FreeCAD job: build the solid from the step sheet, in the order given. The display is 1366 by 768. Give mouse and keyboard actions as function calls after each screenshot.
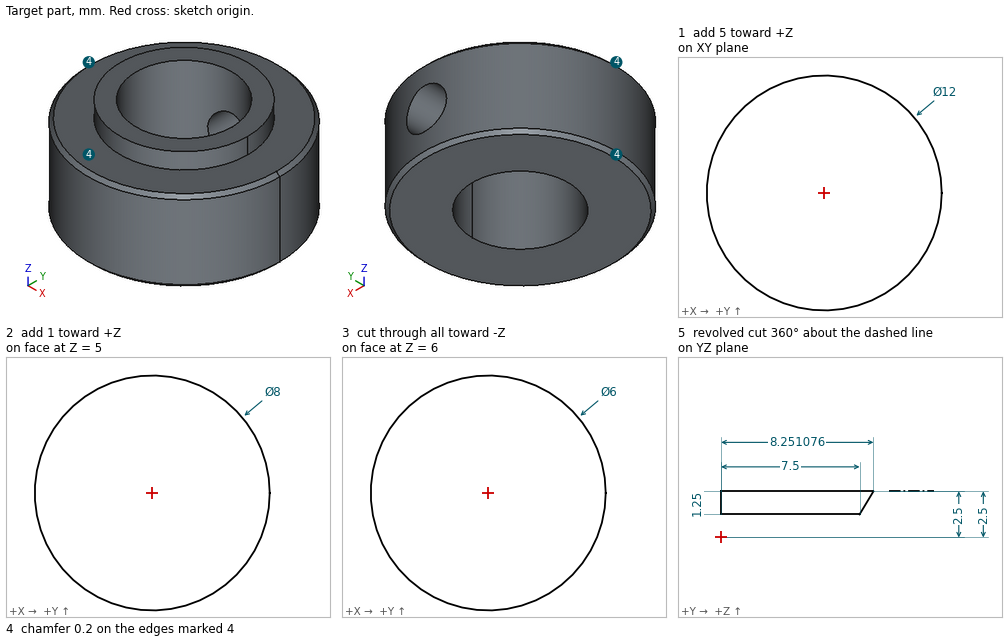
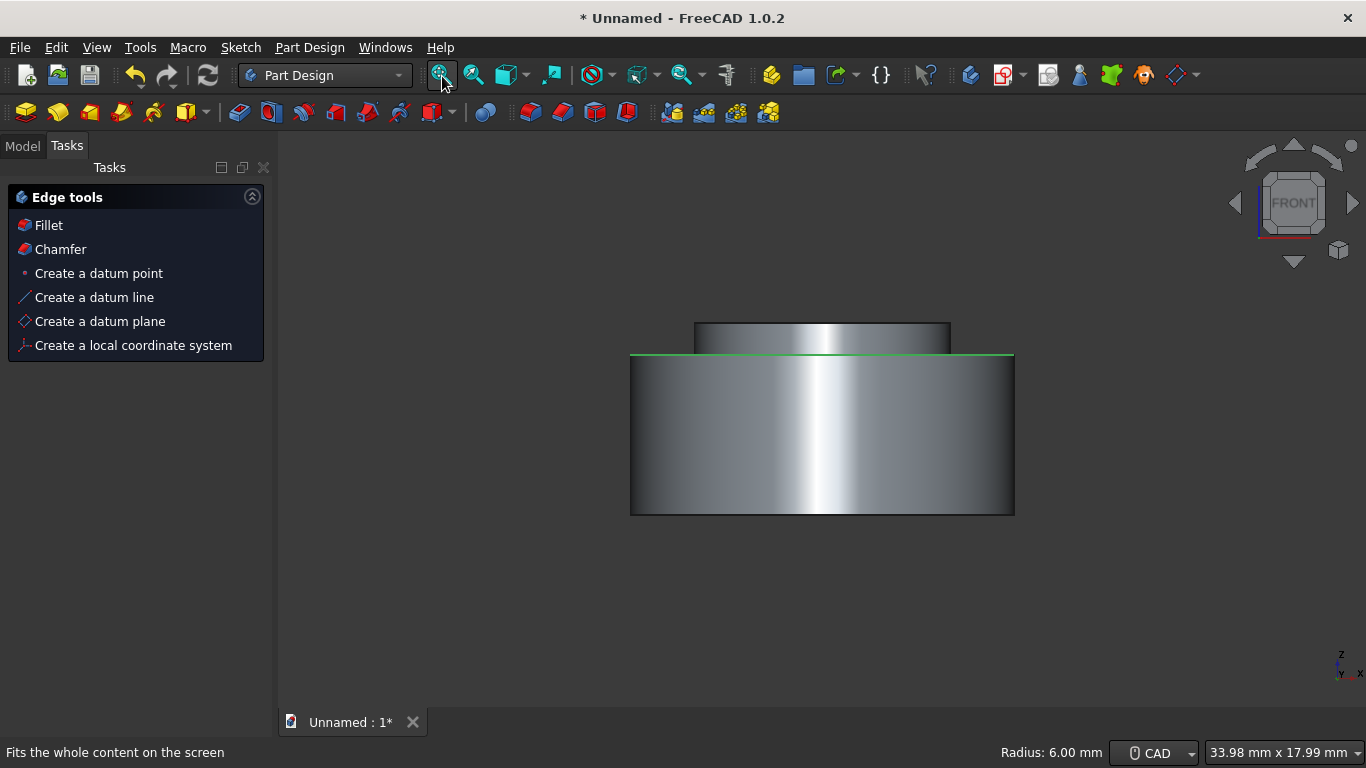
click(666, 514, ctrl)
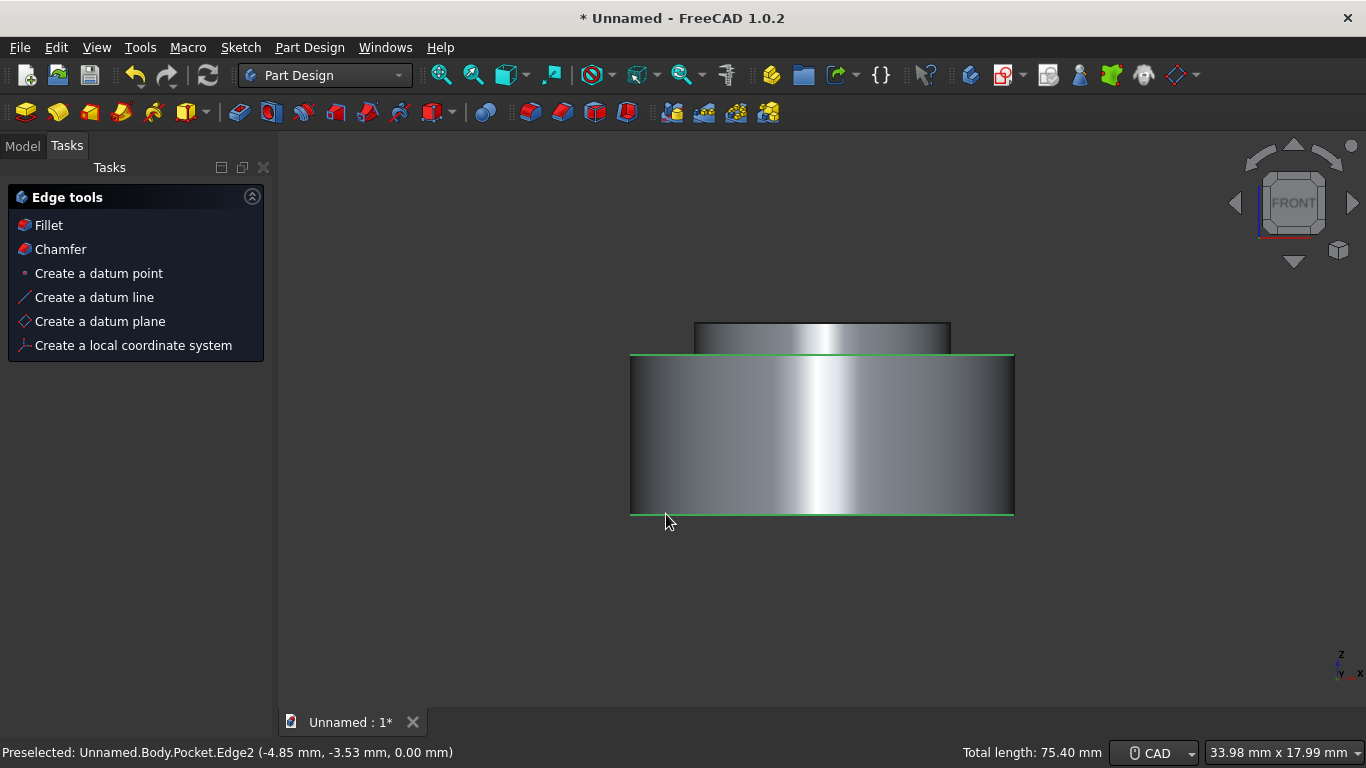
click(564, 112)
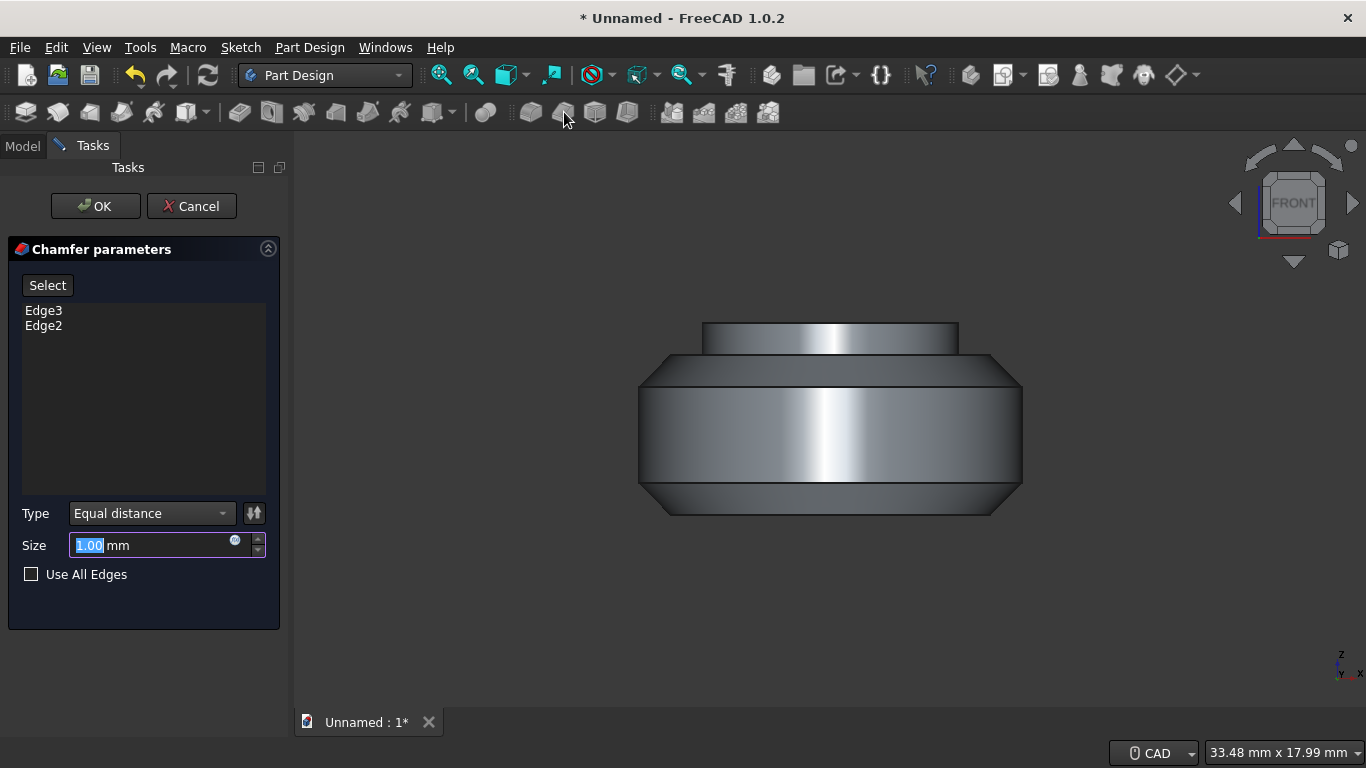
text(0.2)
key(Tab)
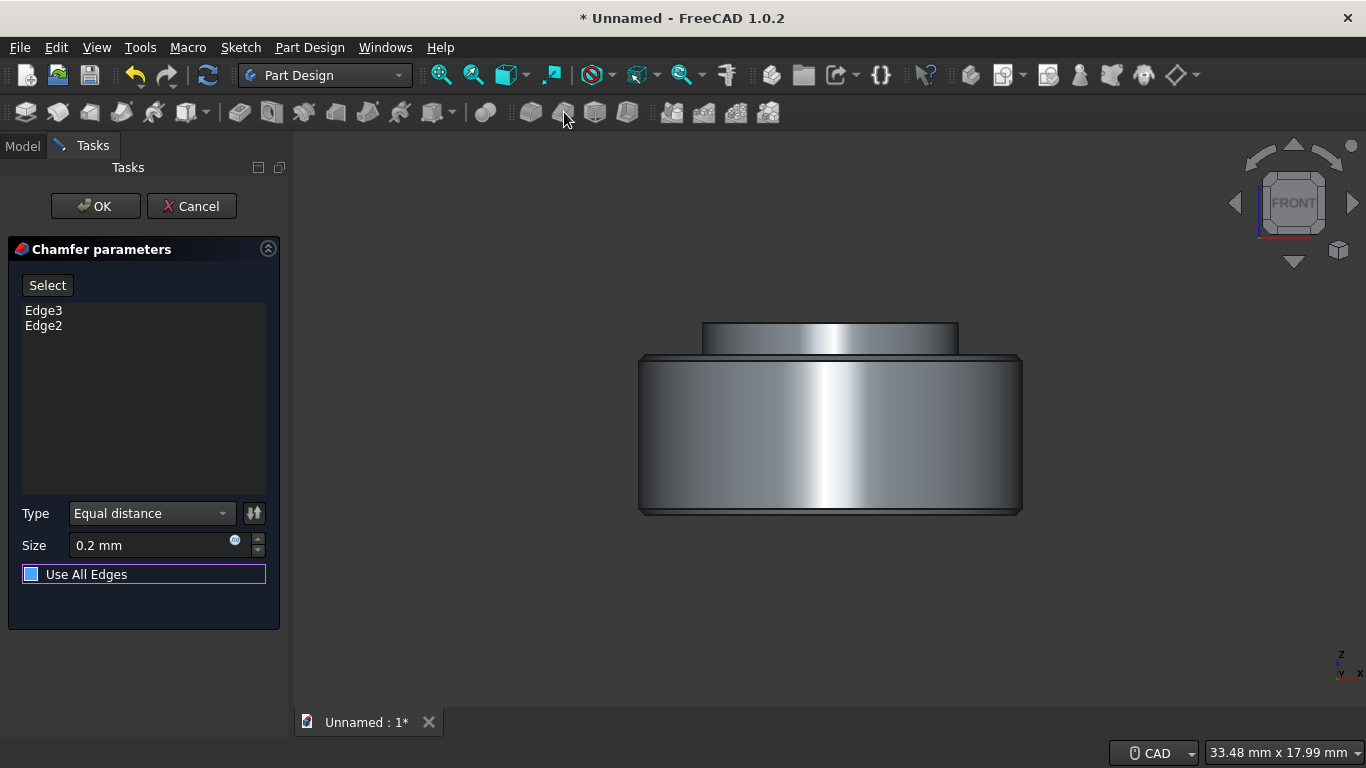
click(96, 206)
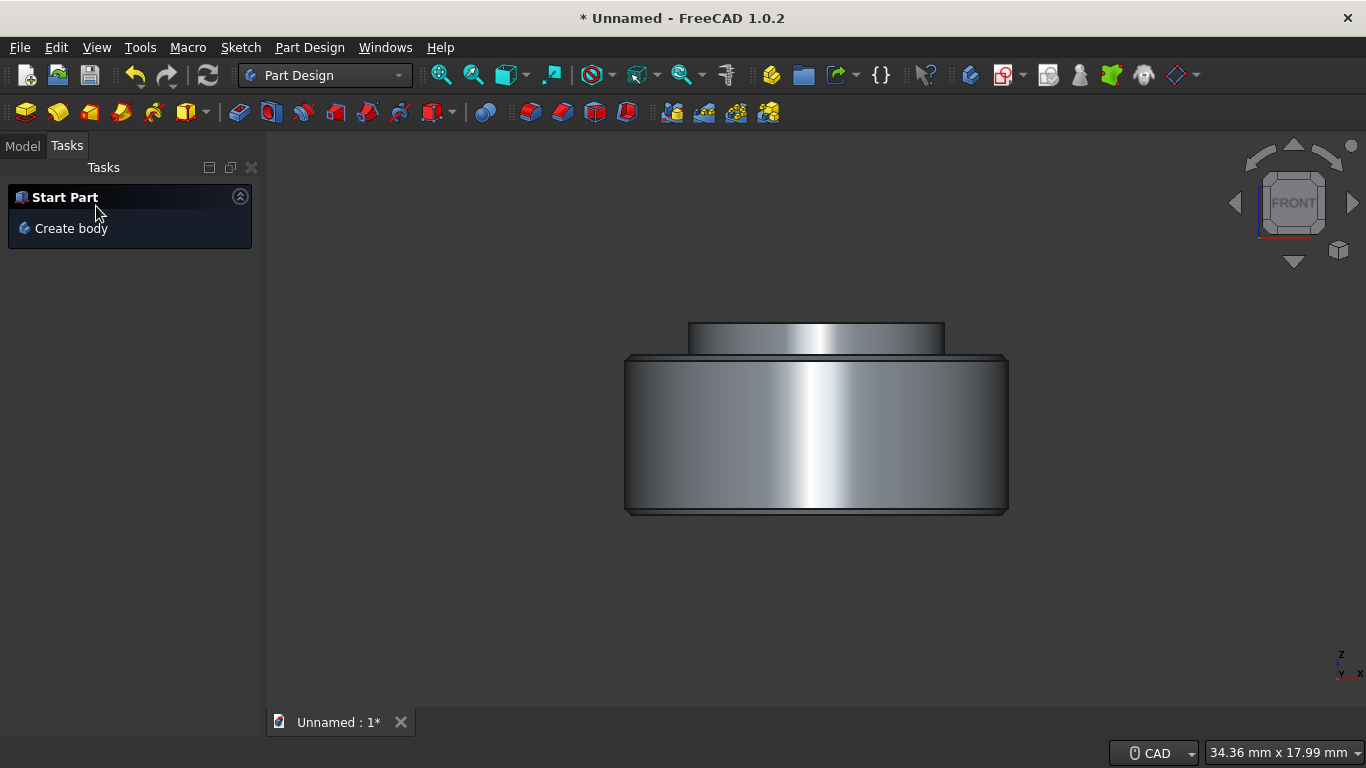
click(442, 76)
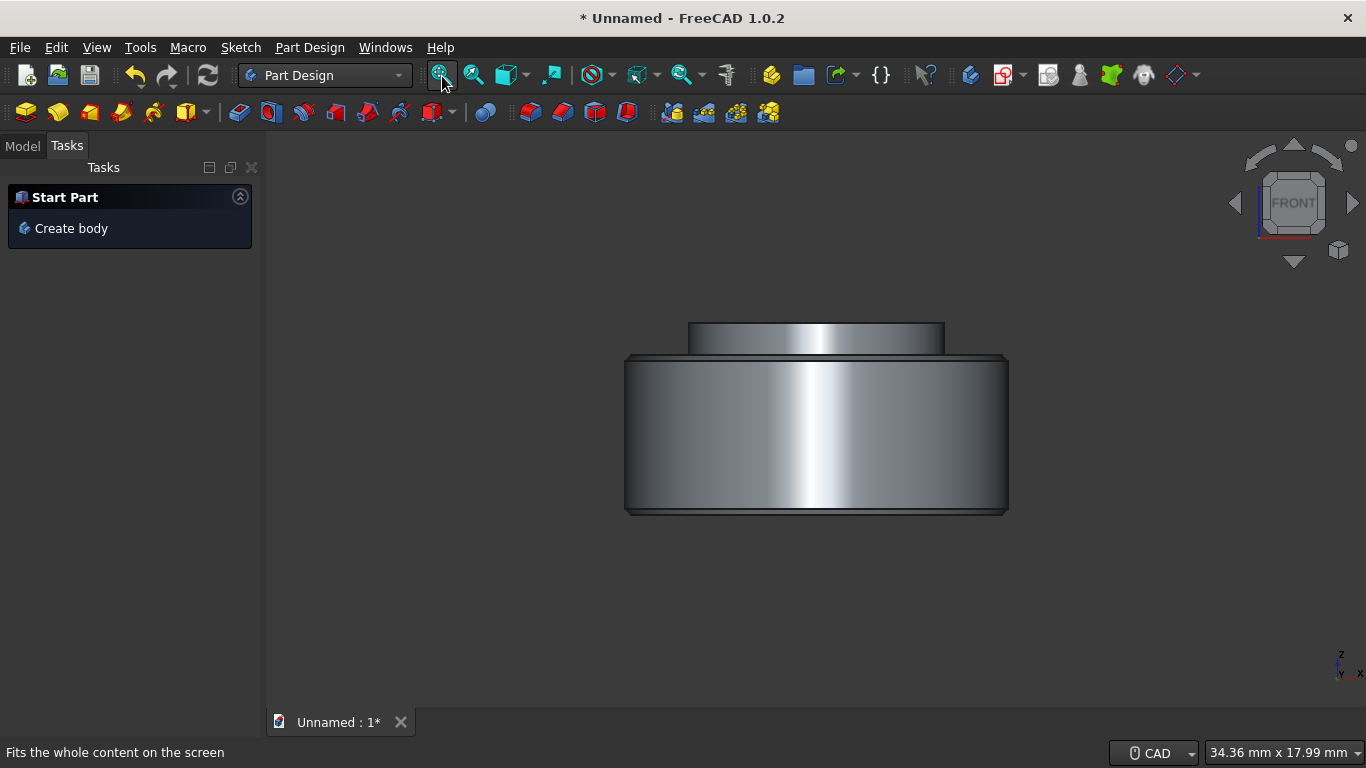
click(1004, 76)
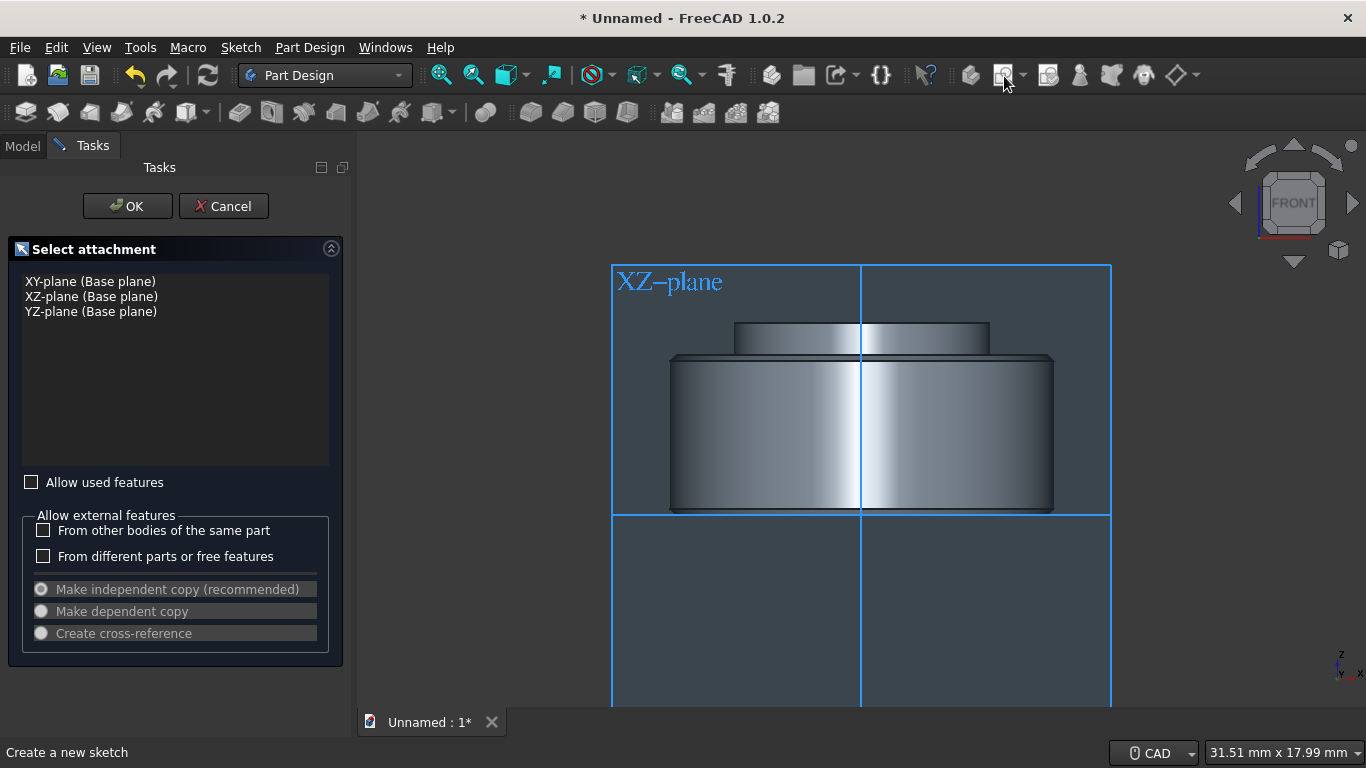
click(82, 312)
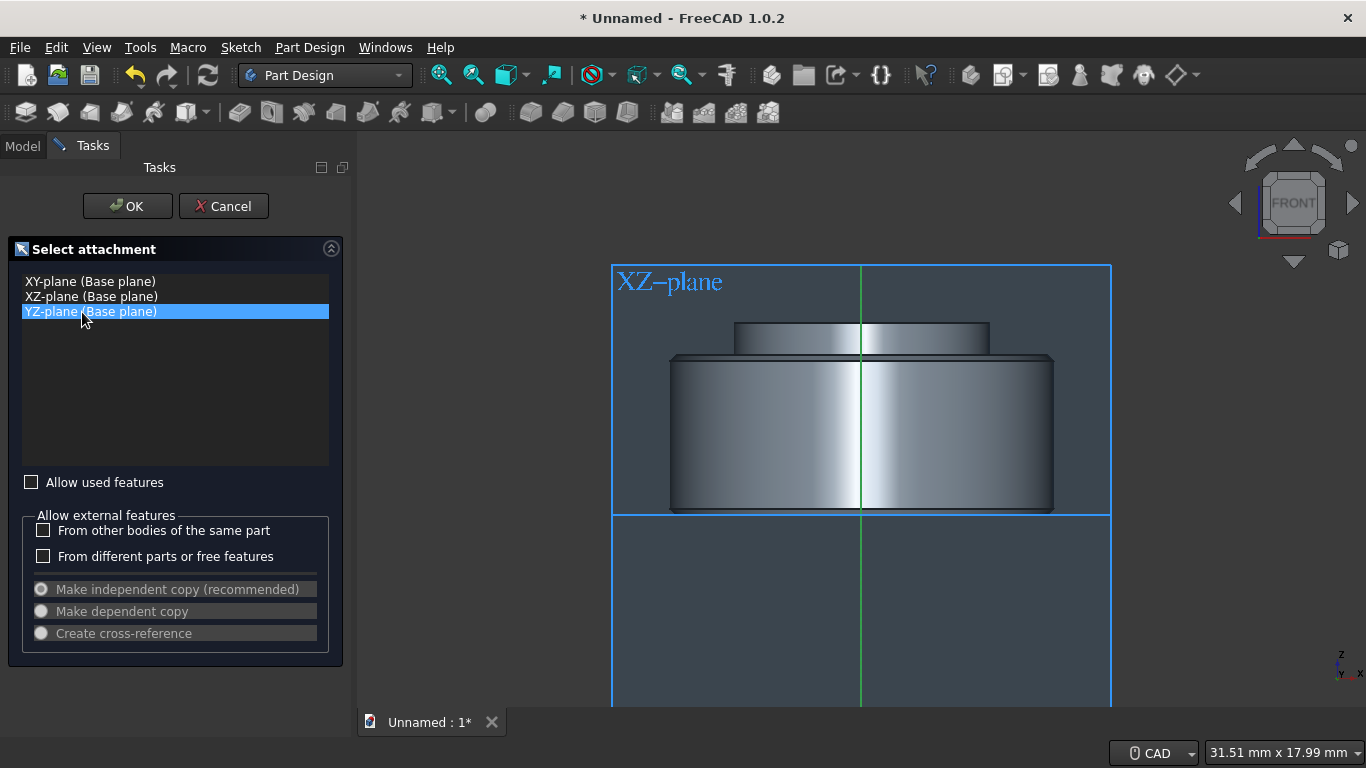
click(128, 206)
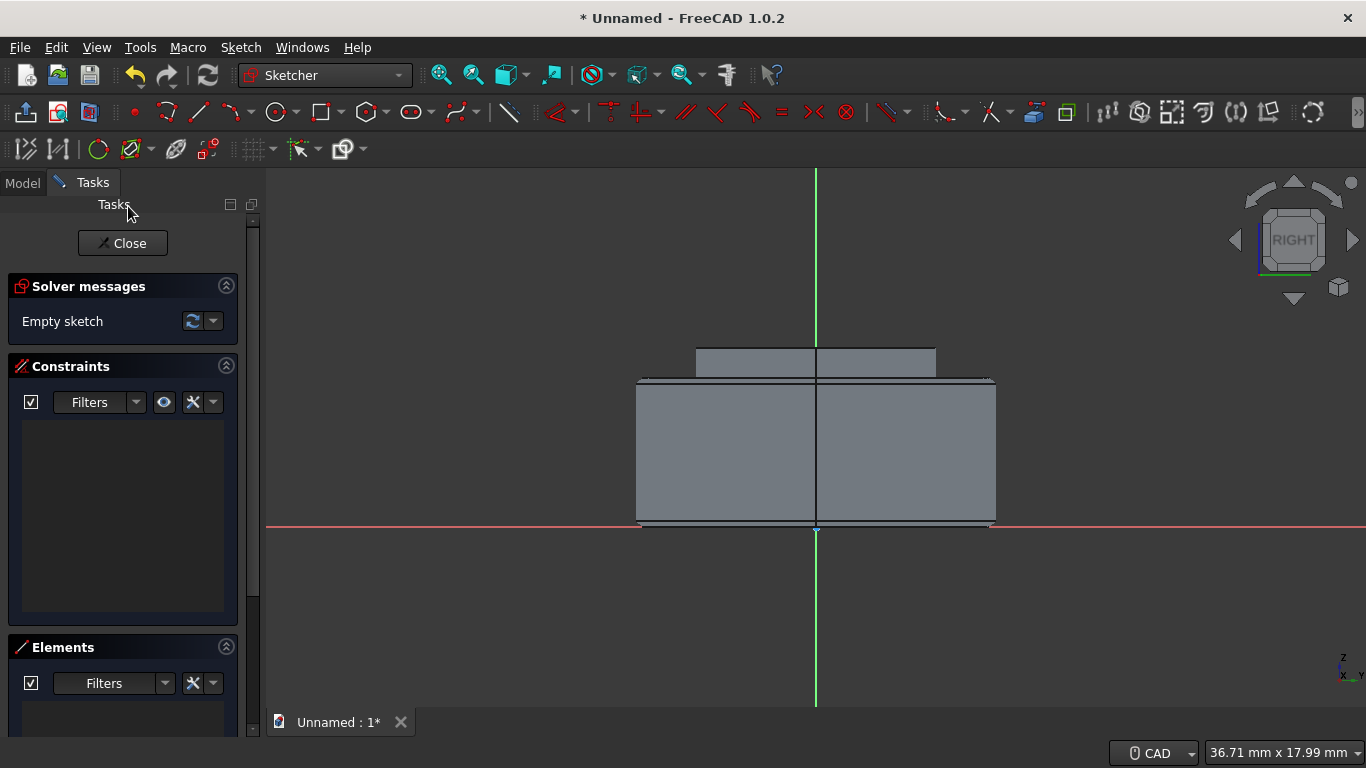
click(90, 112)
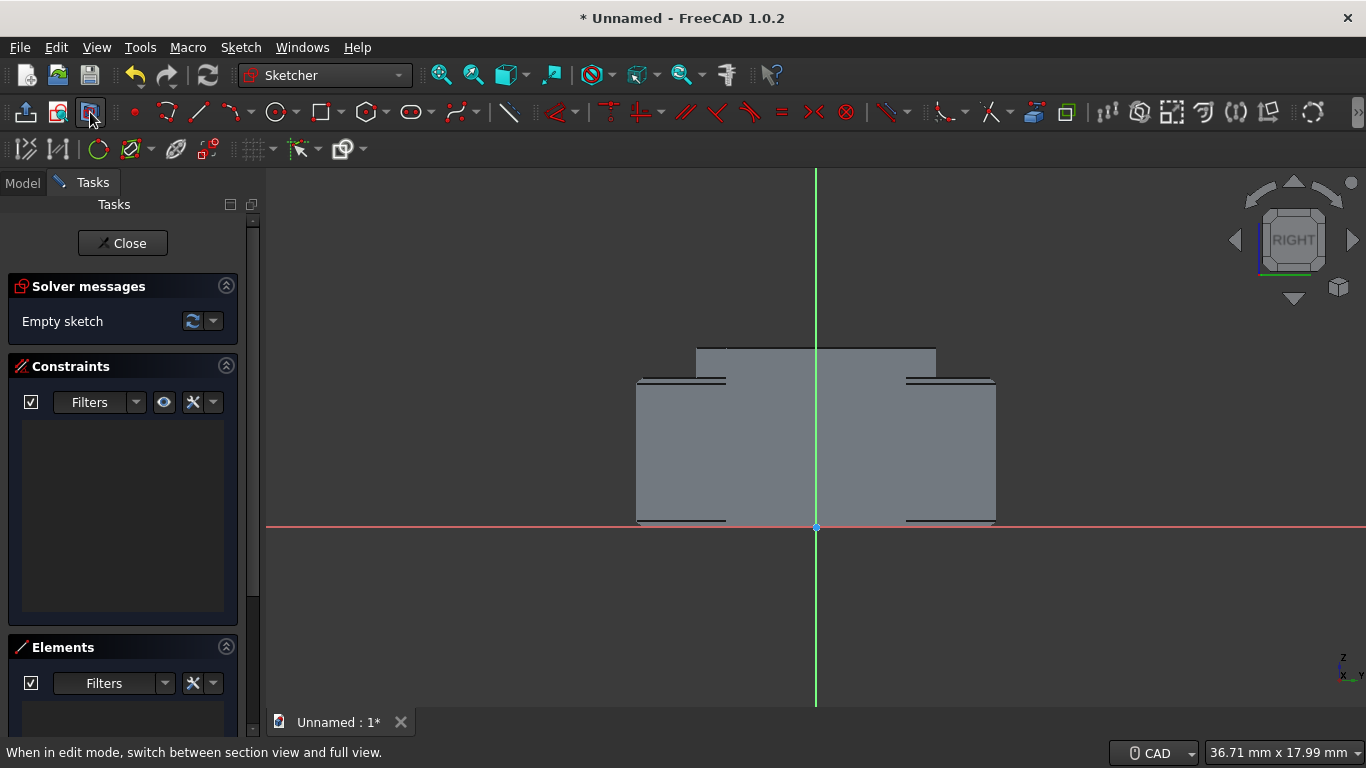
scroll(1201, 554, up, 3)